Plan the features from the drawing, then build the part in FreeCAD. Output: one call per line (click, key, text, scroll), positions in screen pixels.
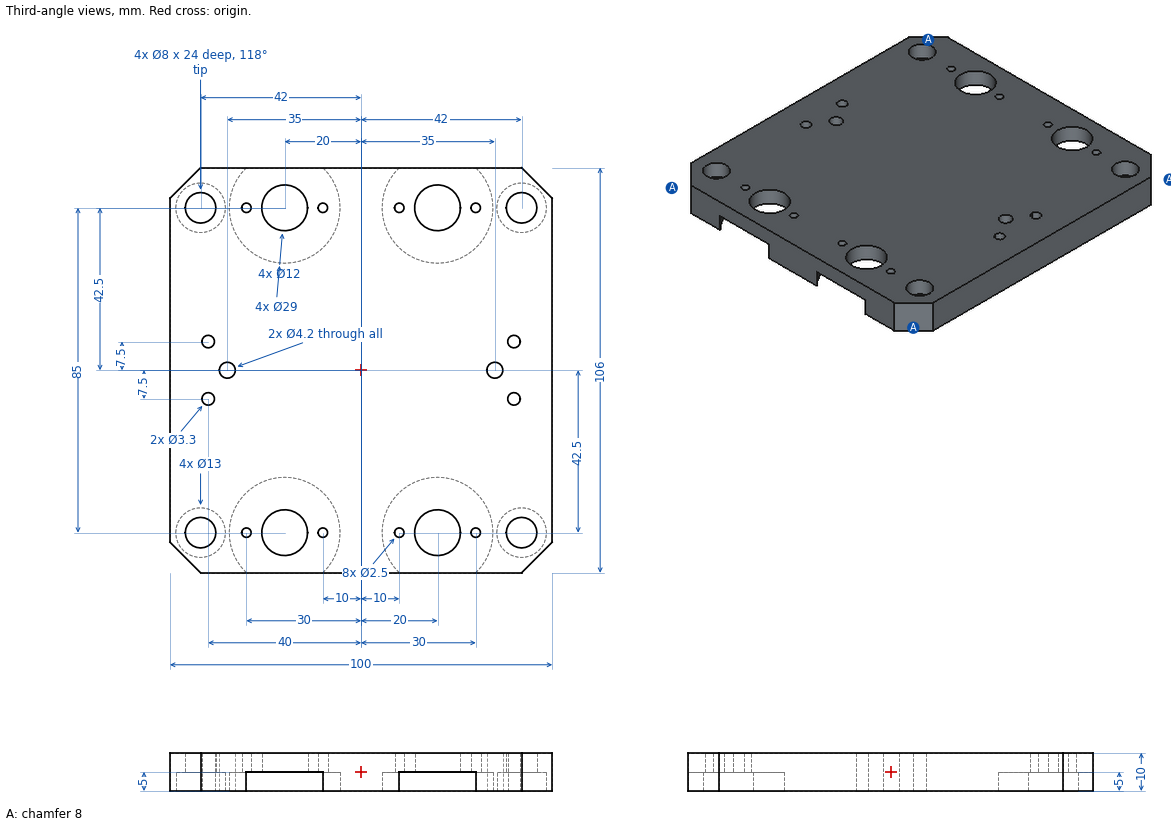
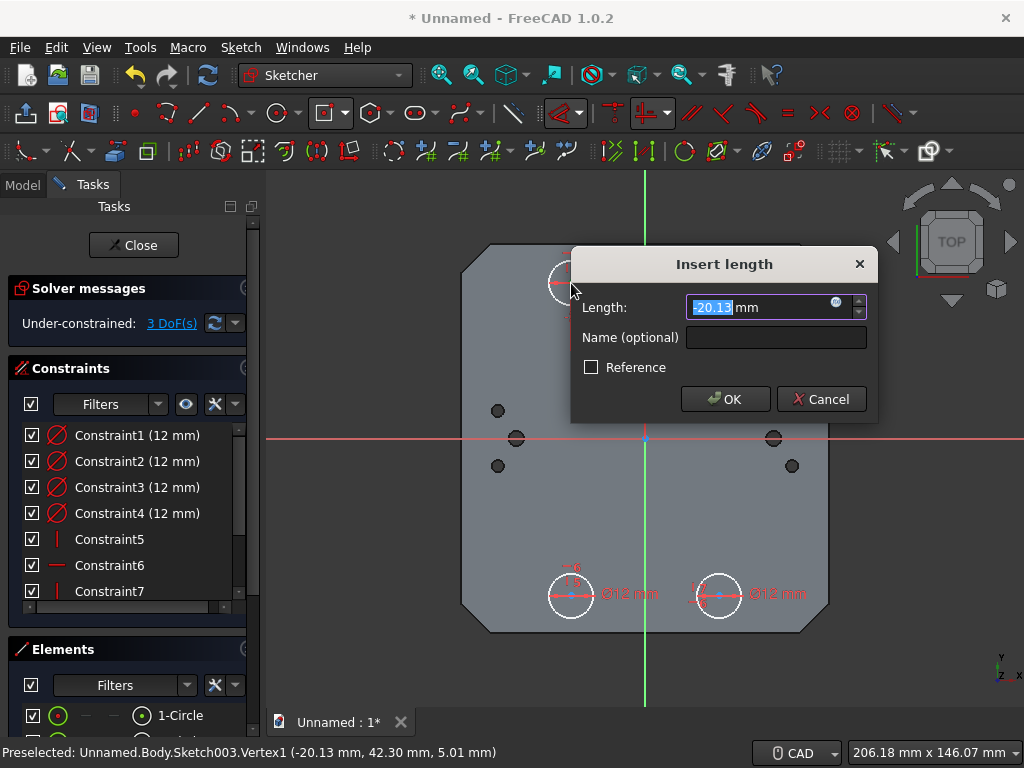
text(-20)
key(Return)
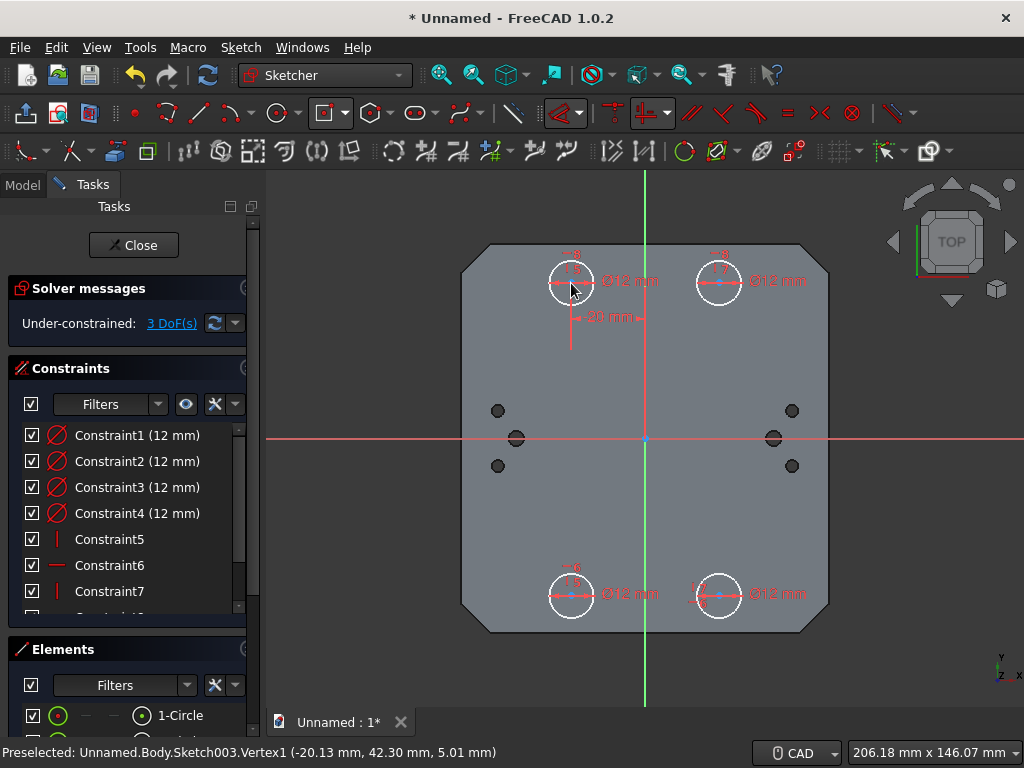
click(719, 596)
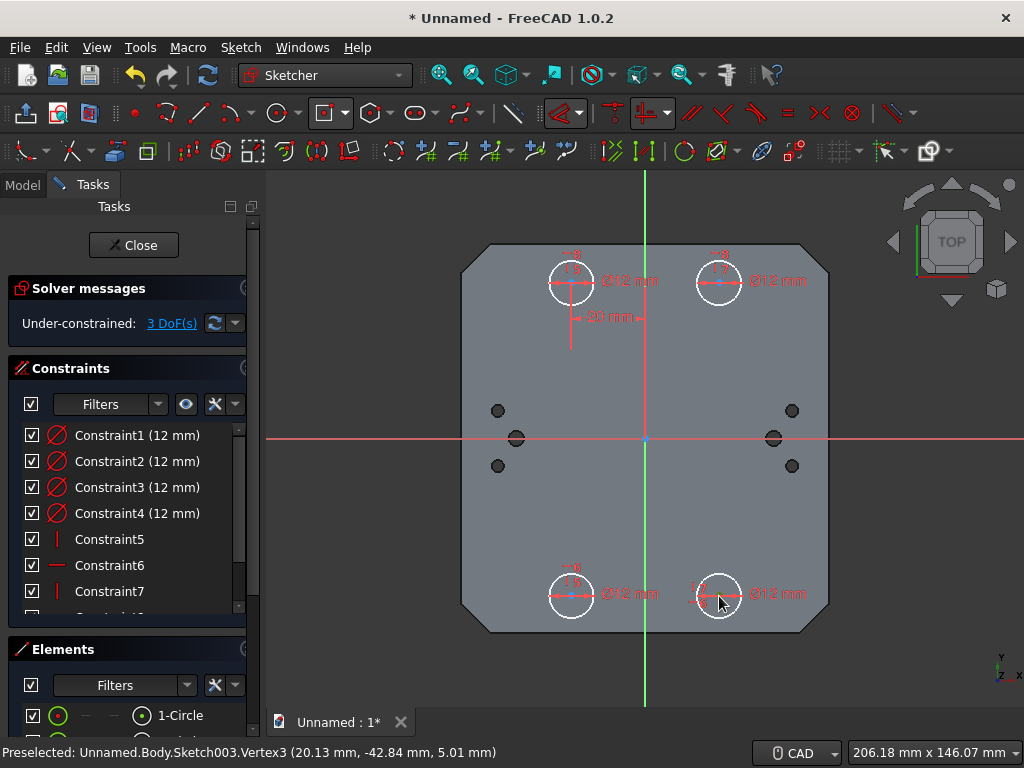
click(582, 114)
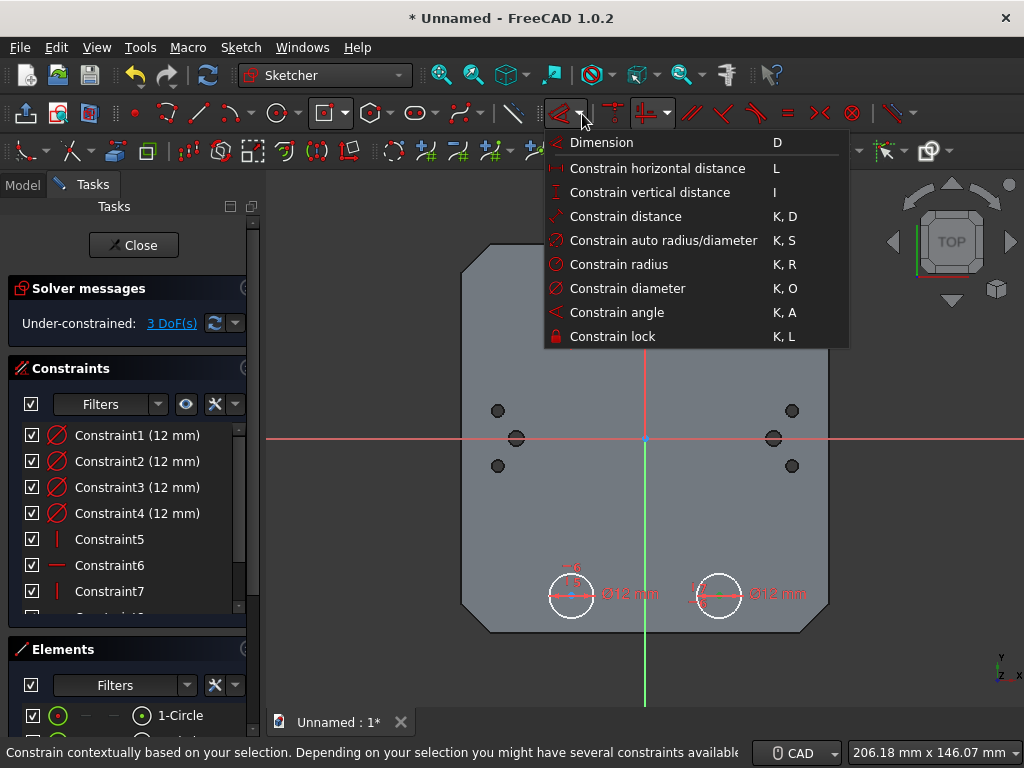
click(697, 168)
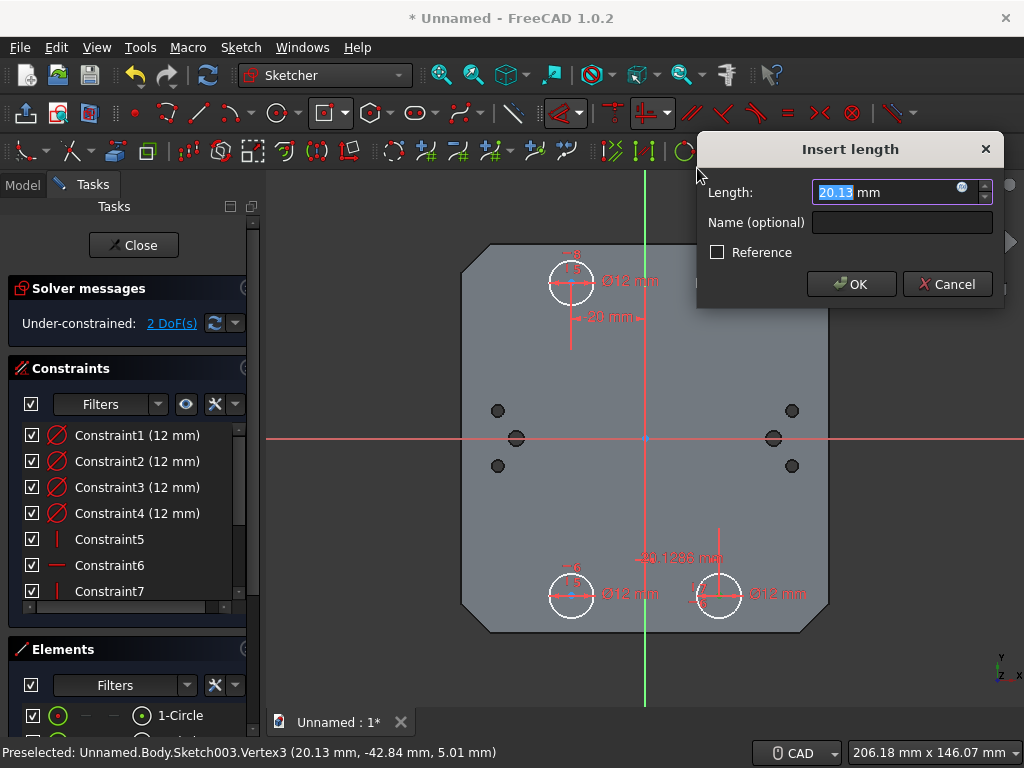
text(20)
key(Return)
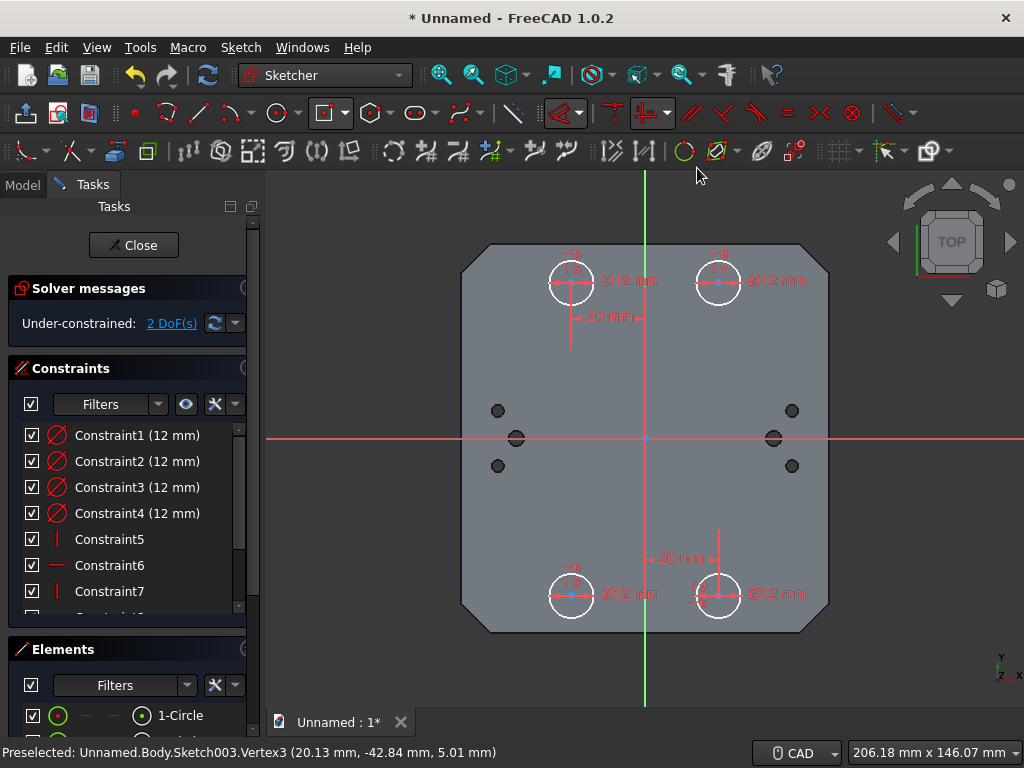
click(571, 283)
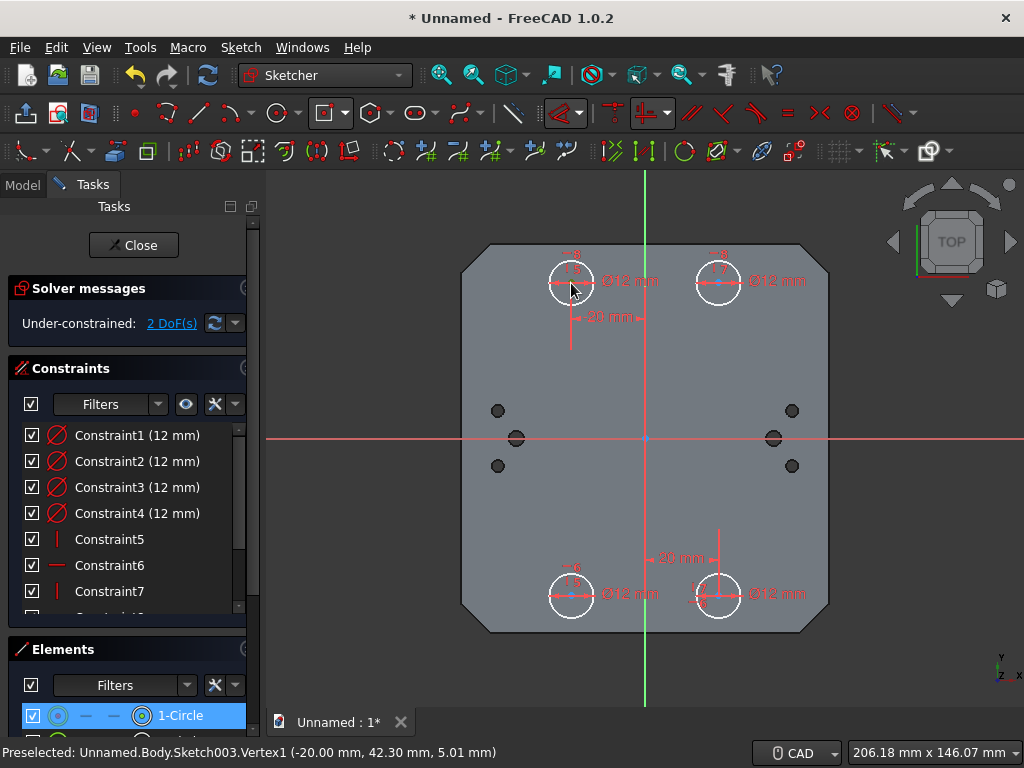
click(571, 596)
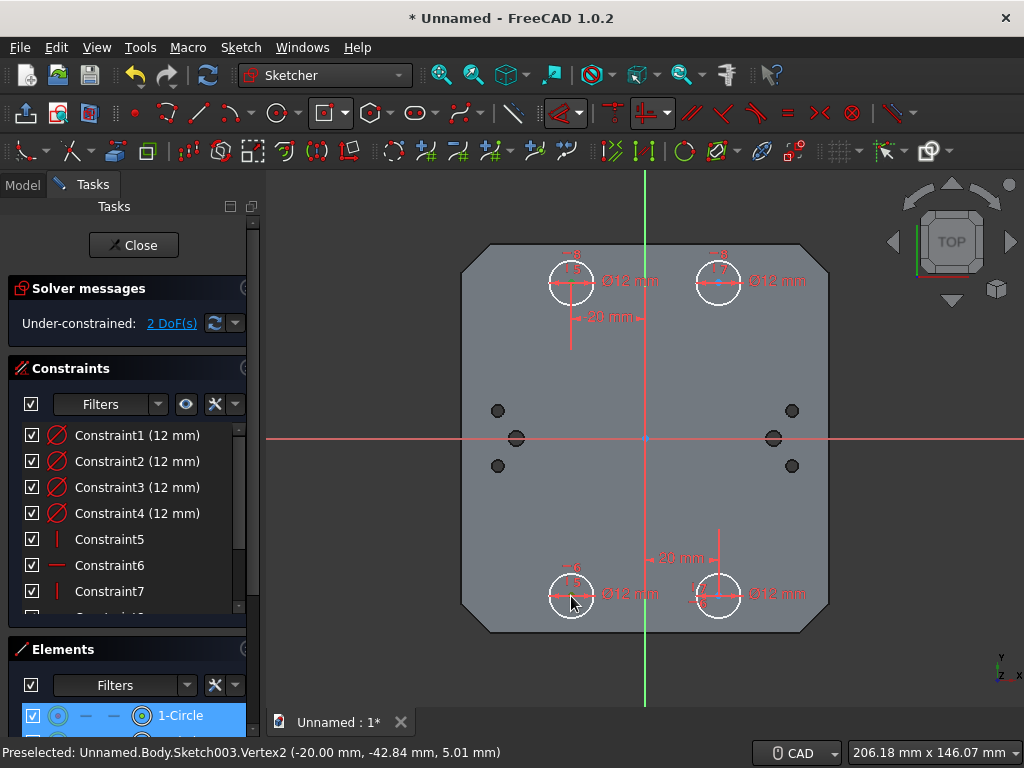
click(582, 114)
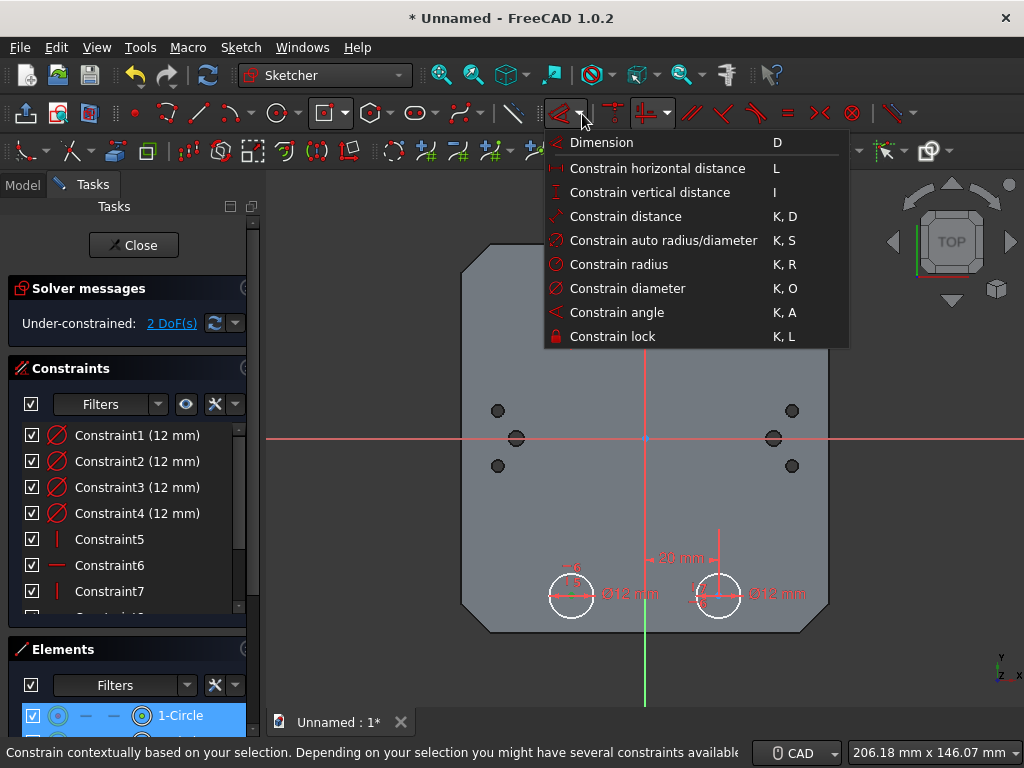
click(697, 192)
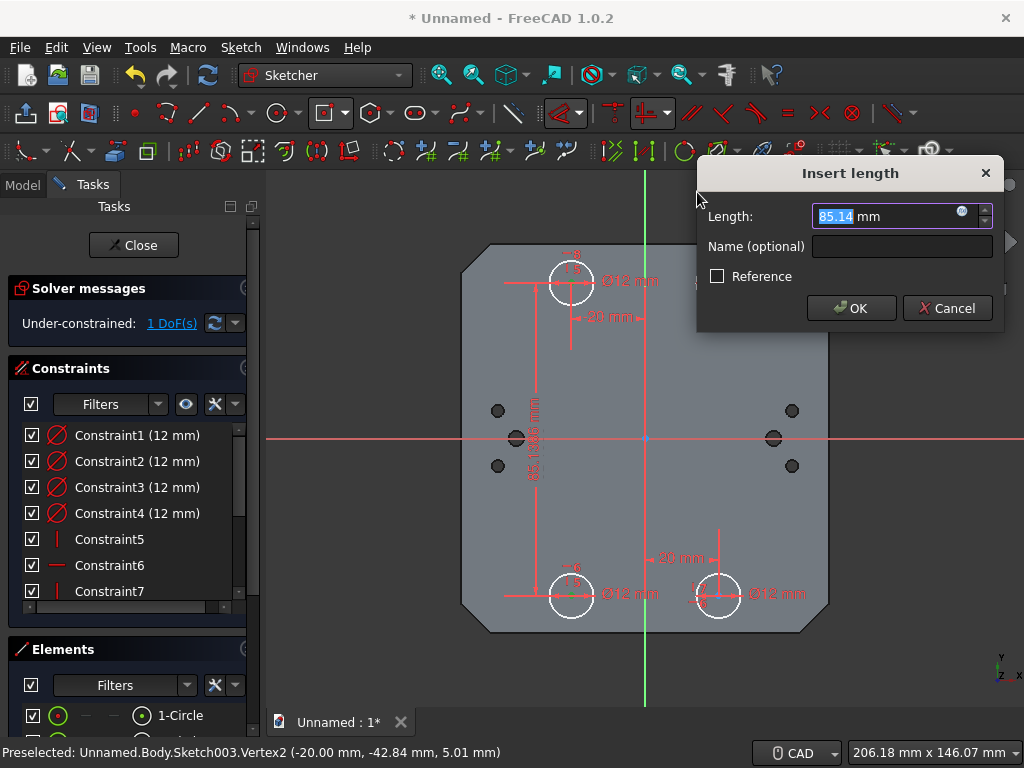
text(85)
key(Return)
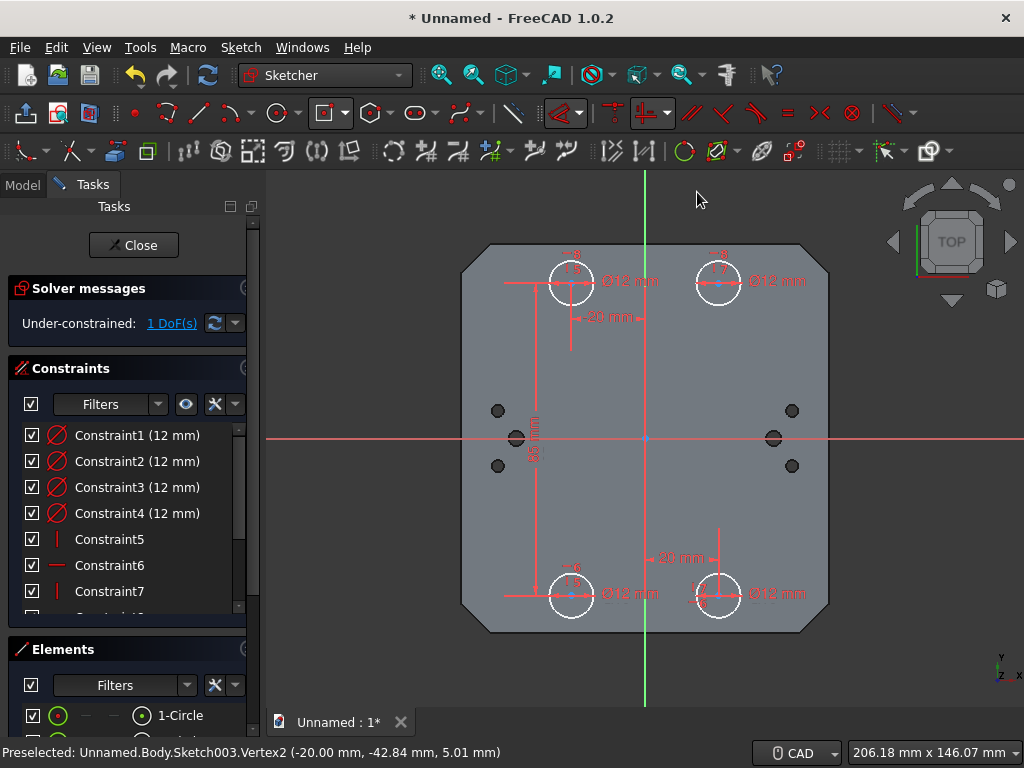
click(571, 283)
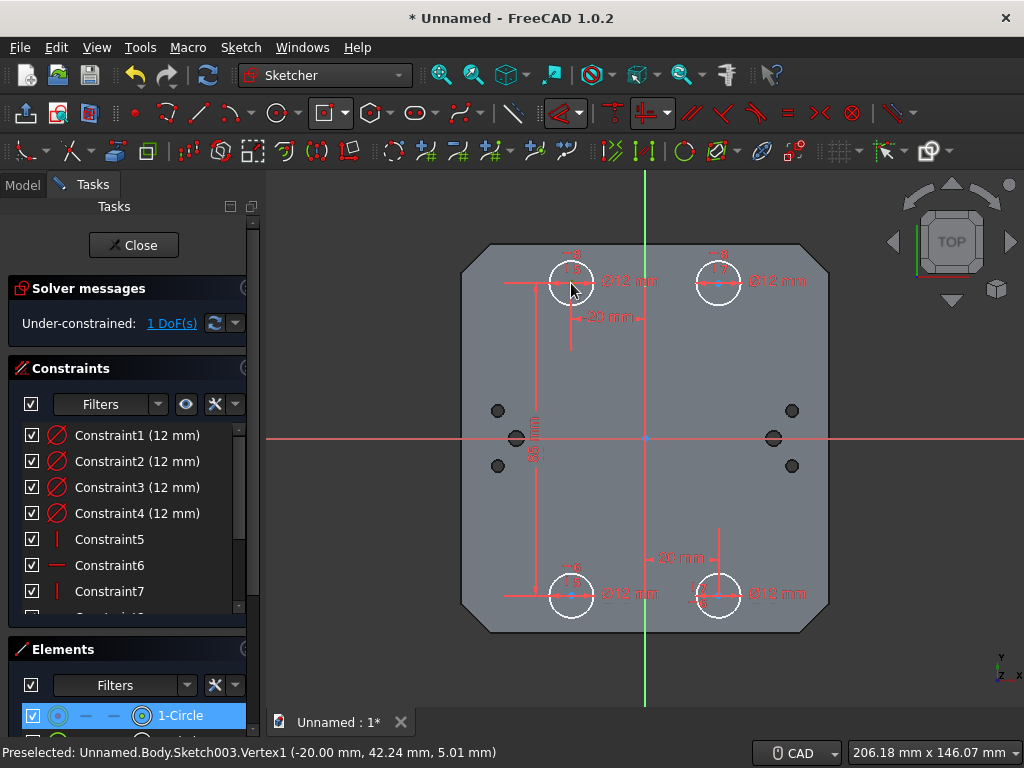
click(582, 114)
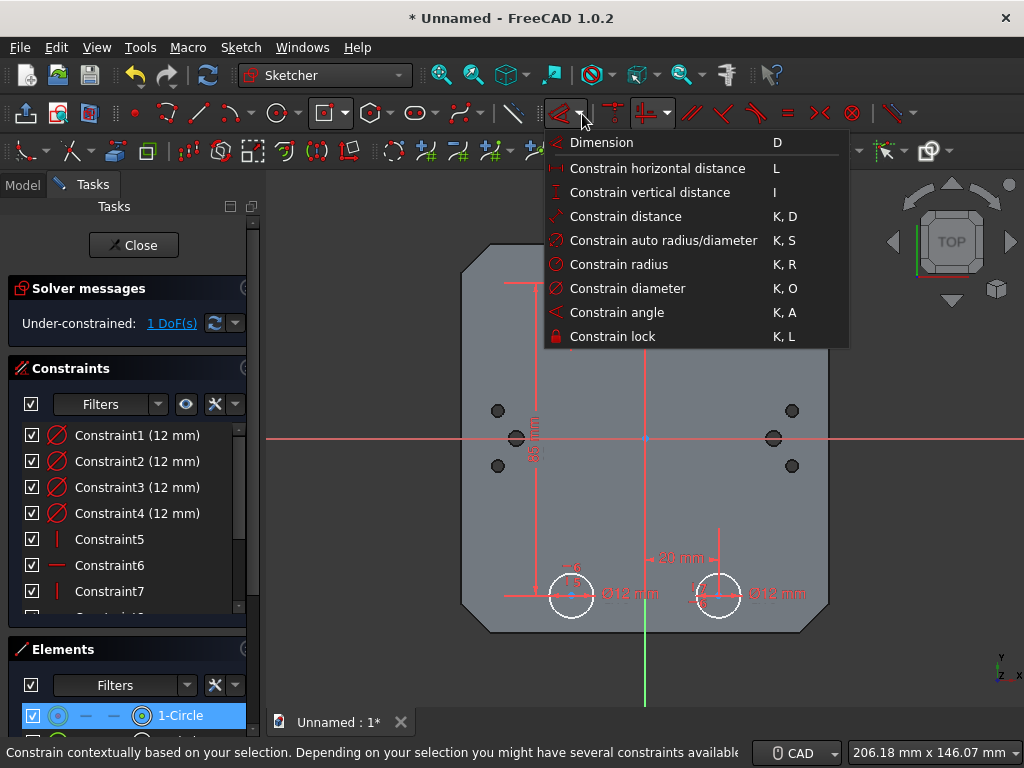
click(697, 192)